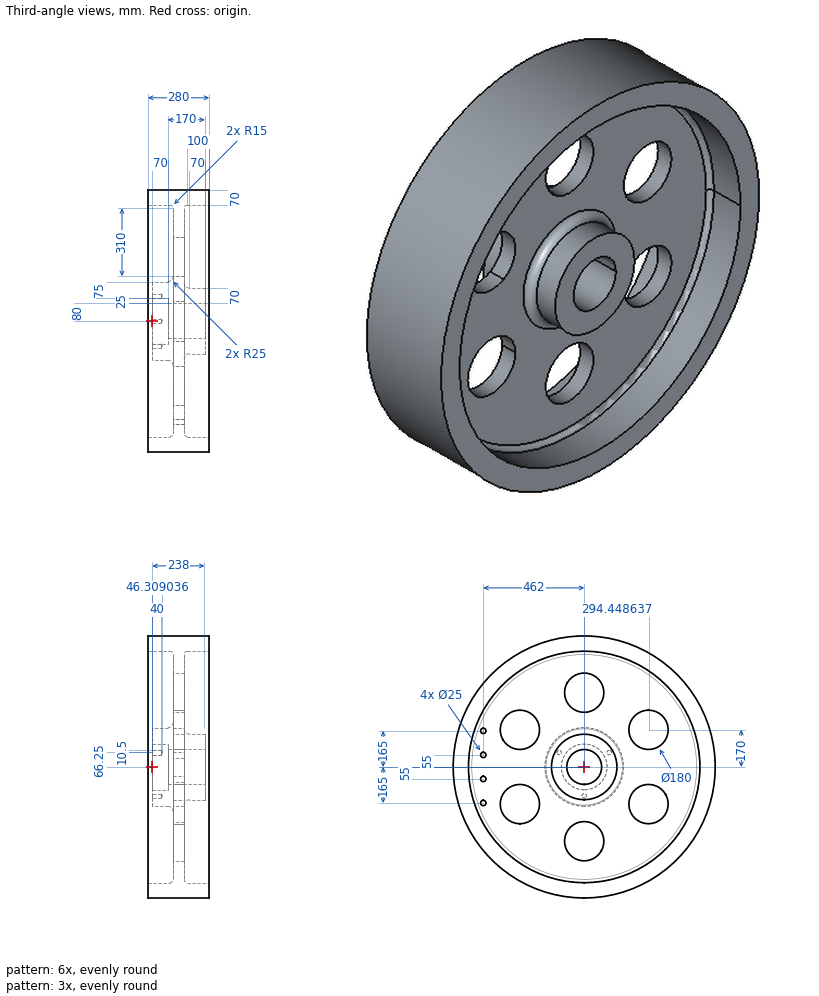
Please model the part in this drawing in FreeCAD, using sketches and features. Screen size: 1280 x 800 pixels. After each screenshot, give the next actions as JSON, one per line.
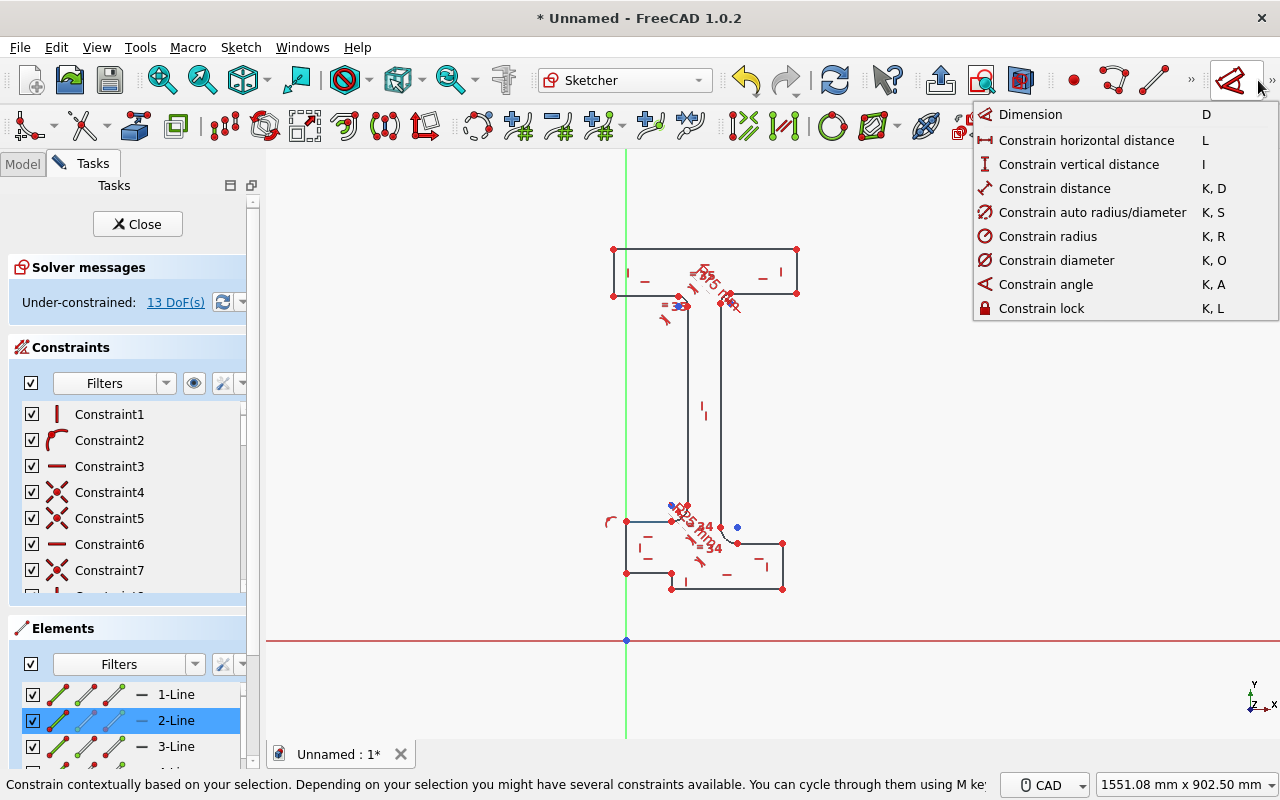
{"action": "left_click", "coordinate": [1126, 140]}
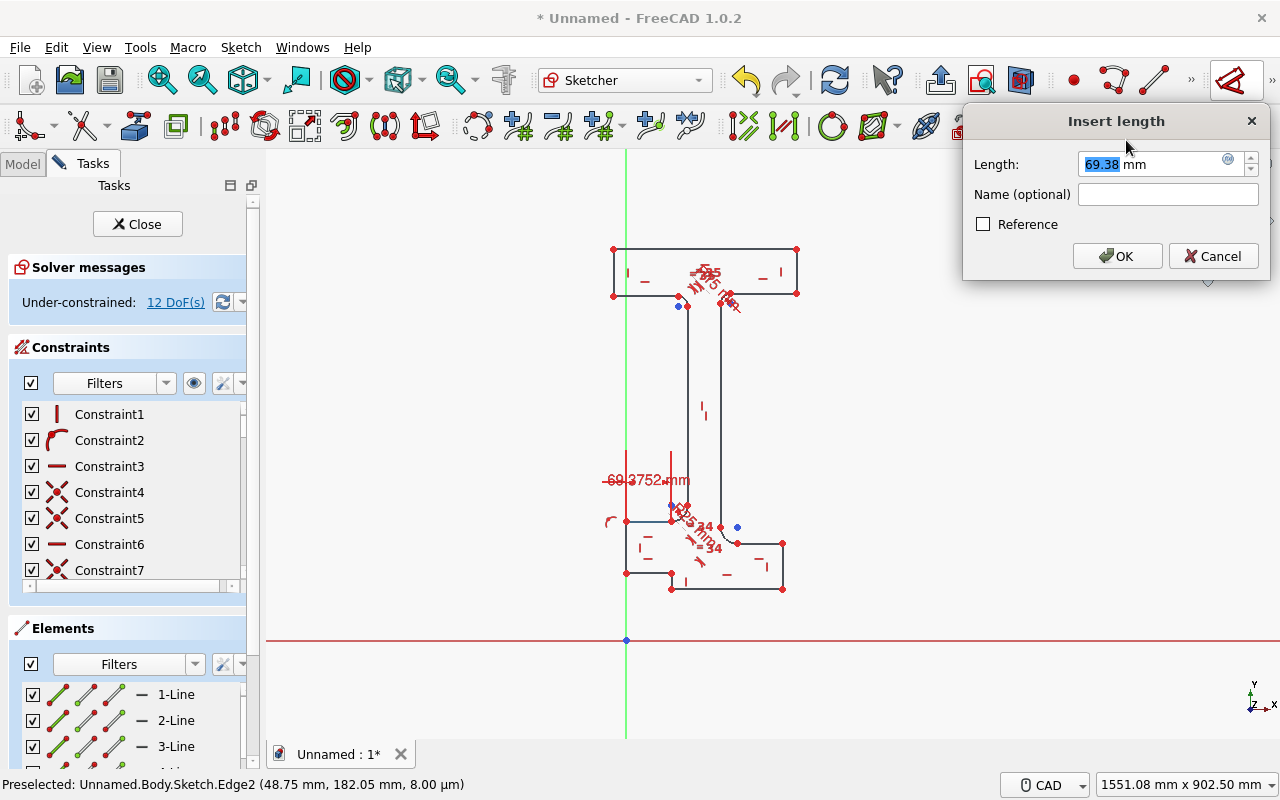
{"action": "type", "text": "70"}
{"action": "key", "text": "Return"}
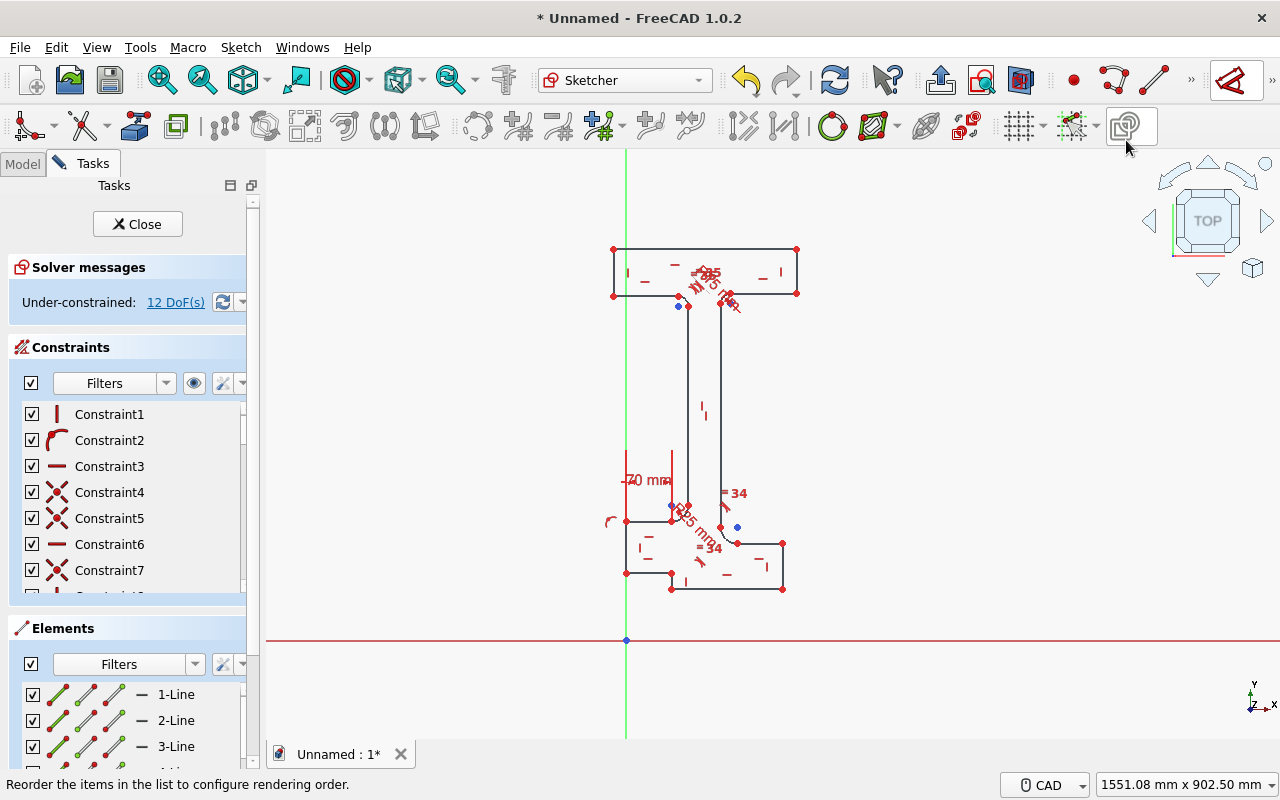
{"action": "left_click", "coordinate": [626, 537]}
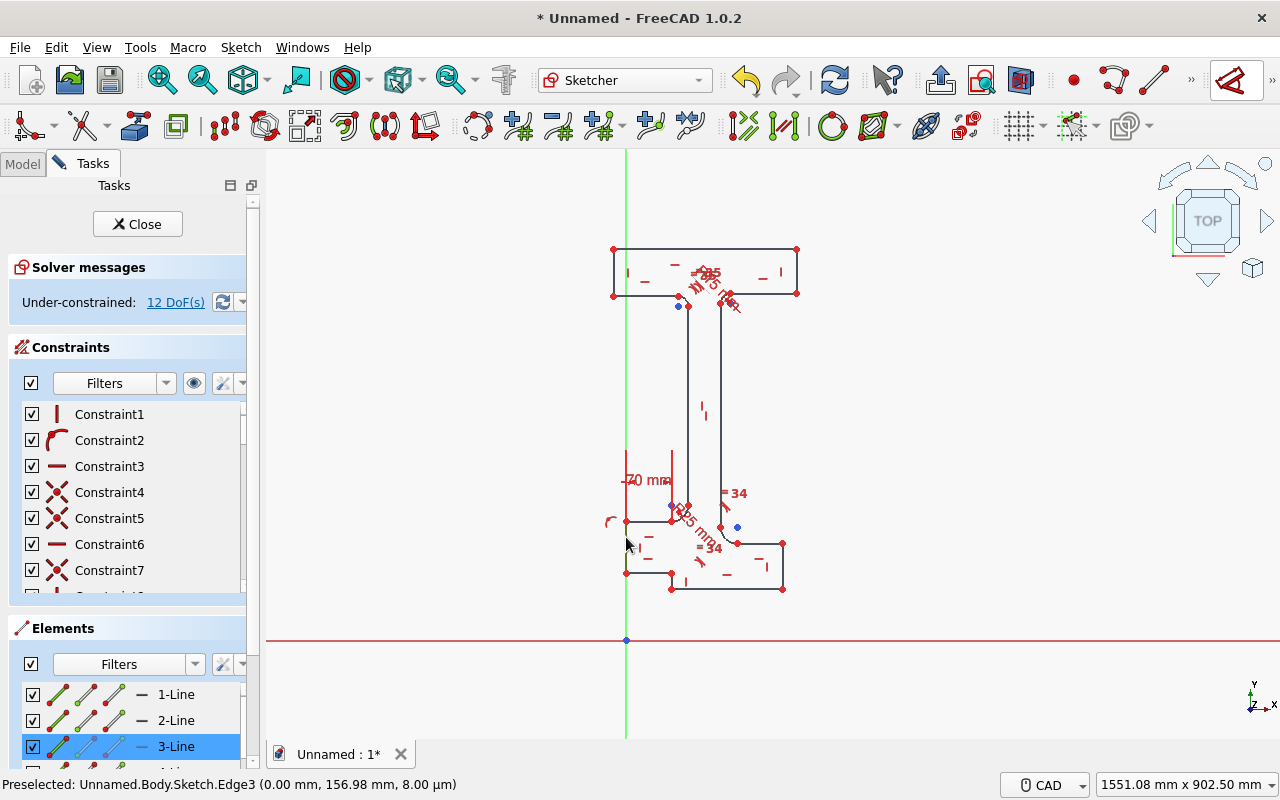
{"action": "key", "text": "i"}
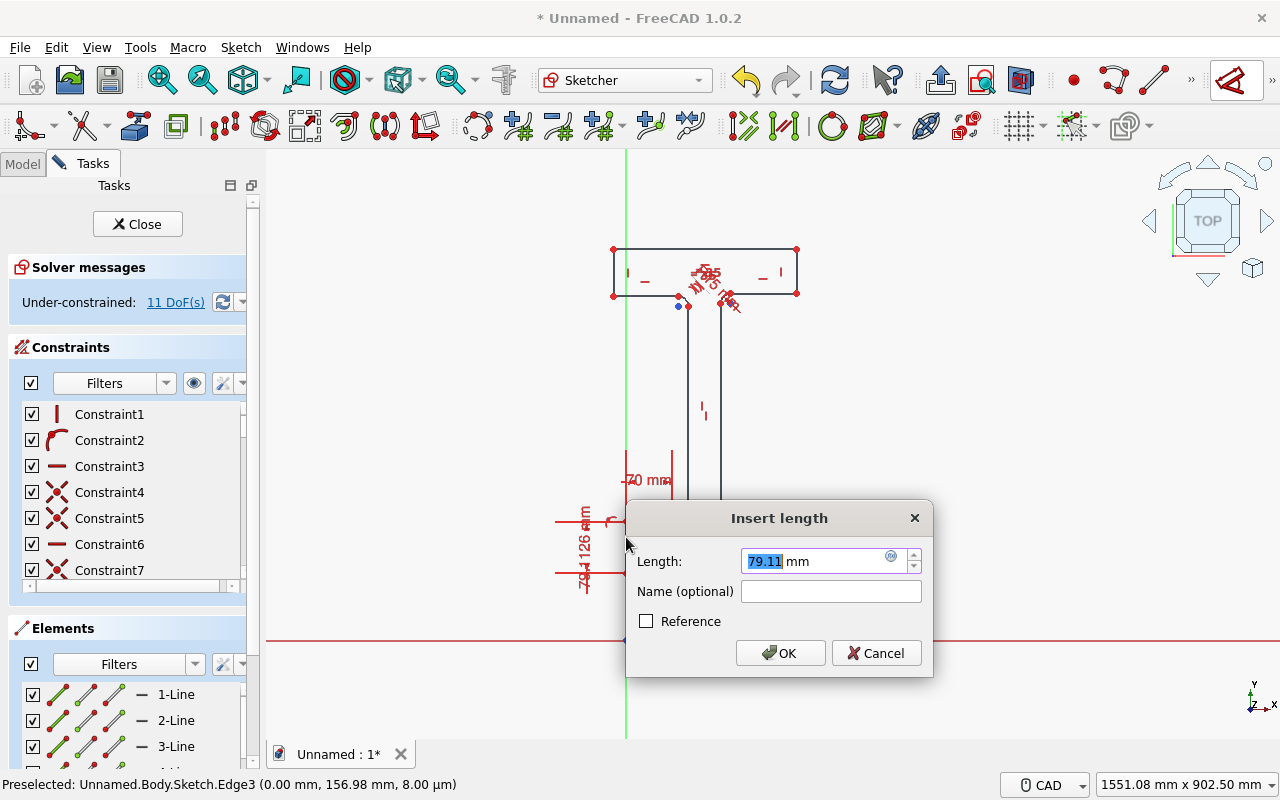
{"action": "type", "text": "75"}
{"action": "key", "text": "Return"}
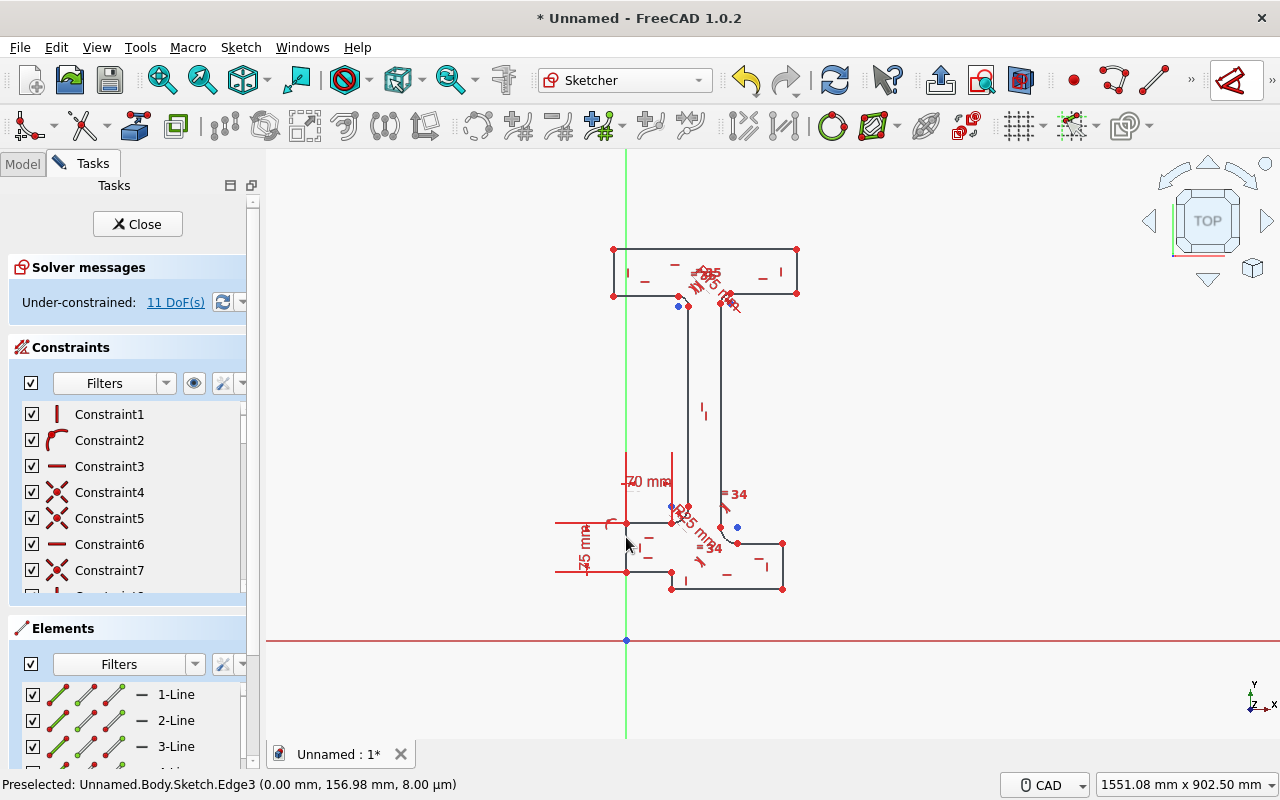
{"action": "left_click", "coordinate": [640, 572]}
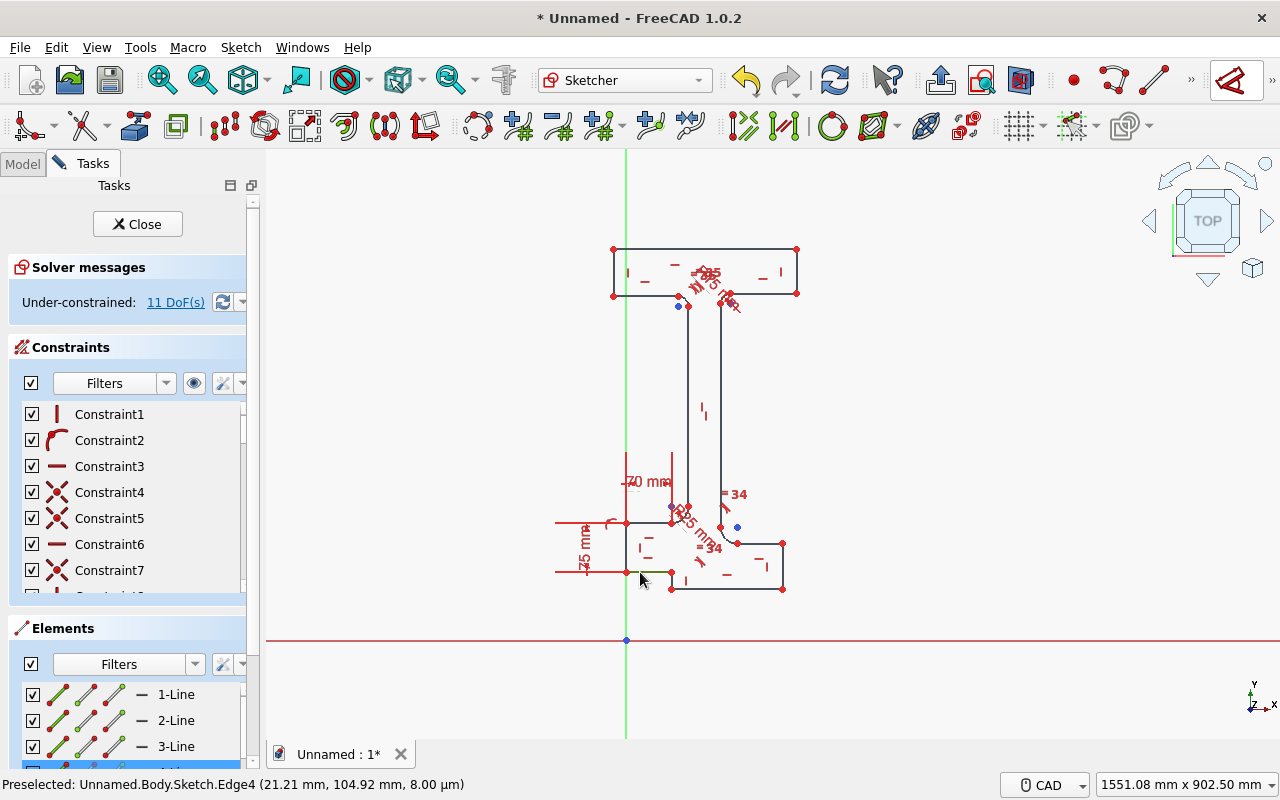
{"action": "key", "text": "l"}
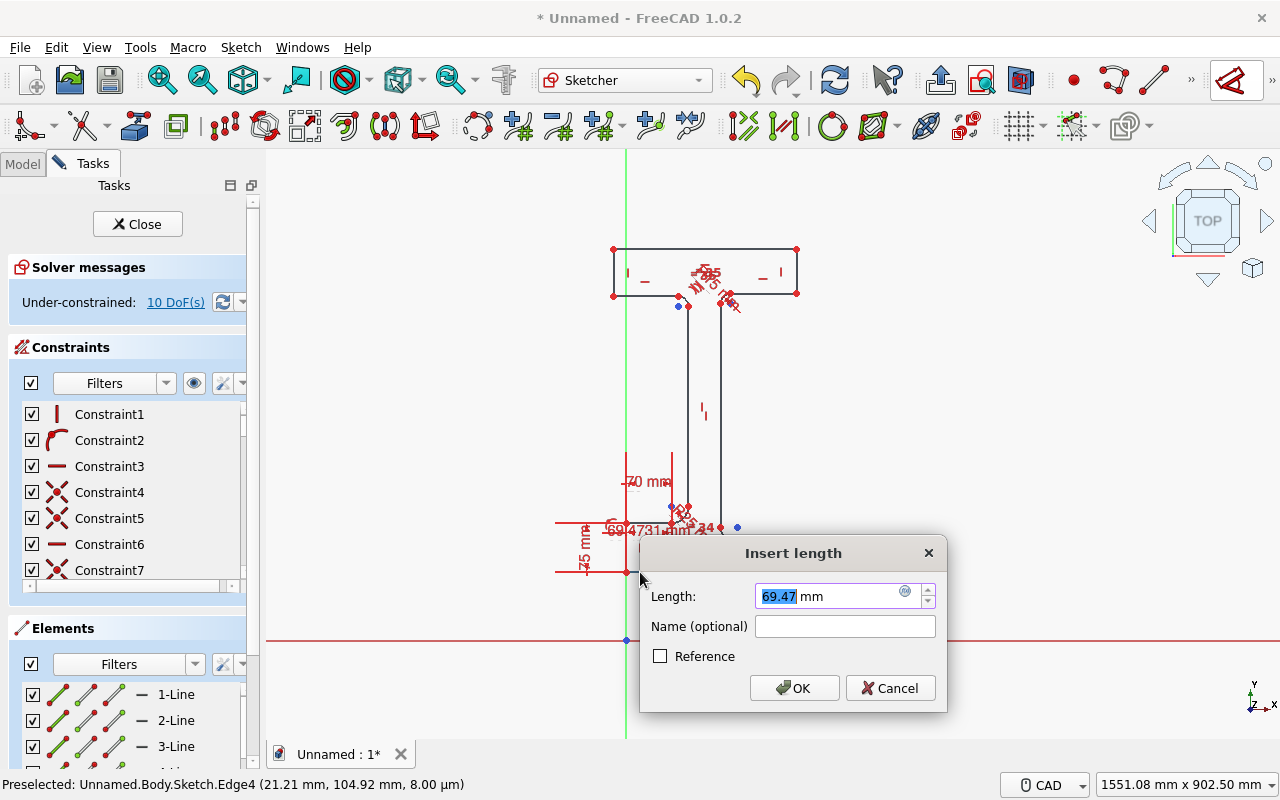
{"action": "type", "text": "70"}
{"action": "key", "text": "Return"}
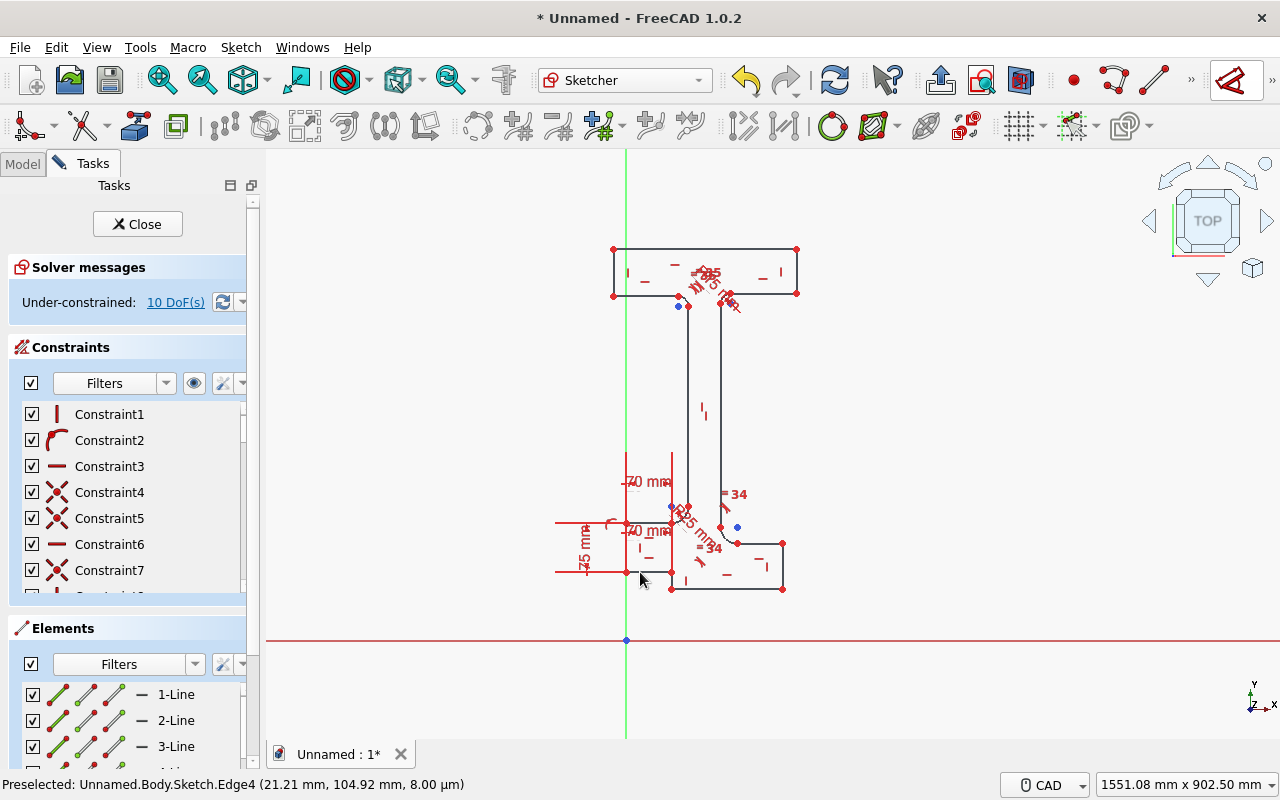
{"action": "scroll", "coordinate": [672, 581], "scroll_direction": "up", "scroll_amount": 5}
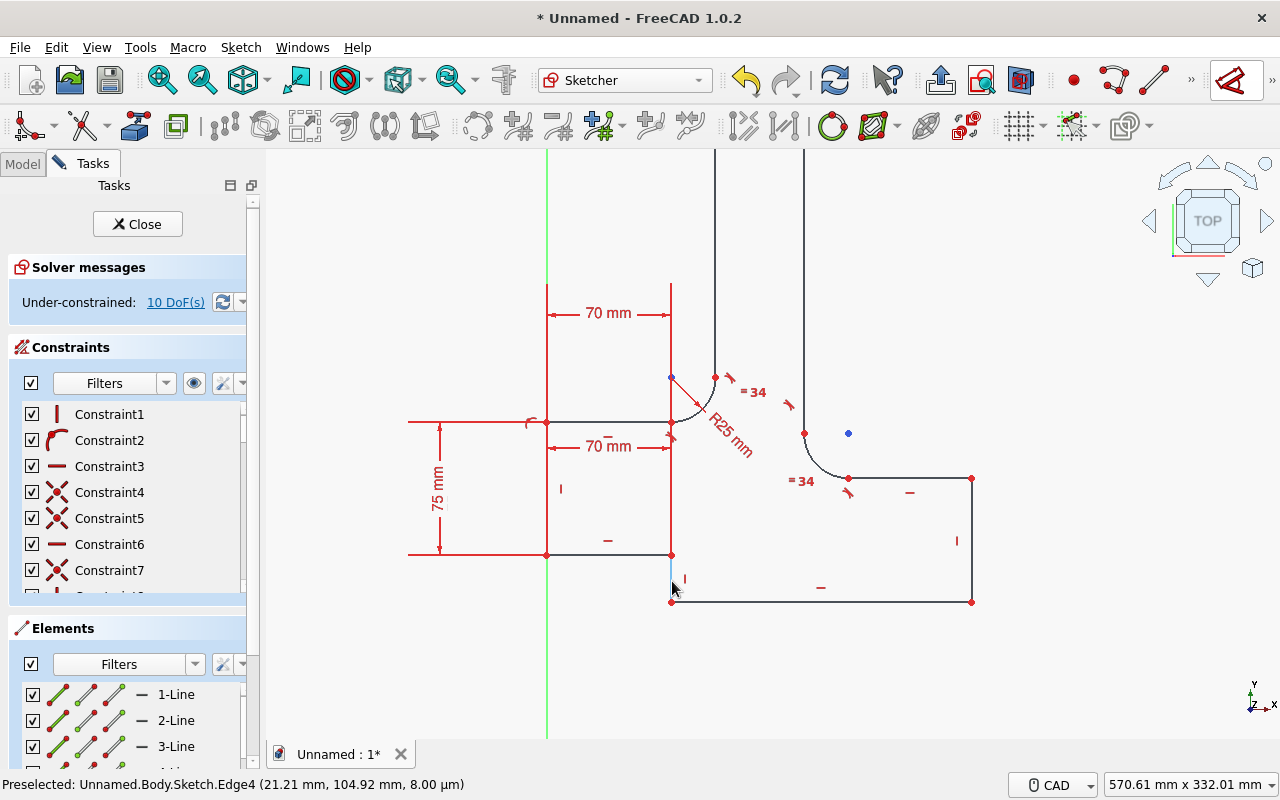
{"action": "left_click", "coordinate": [671, 579]}